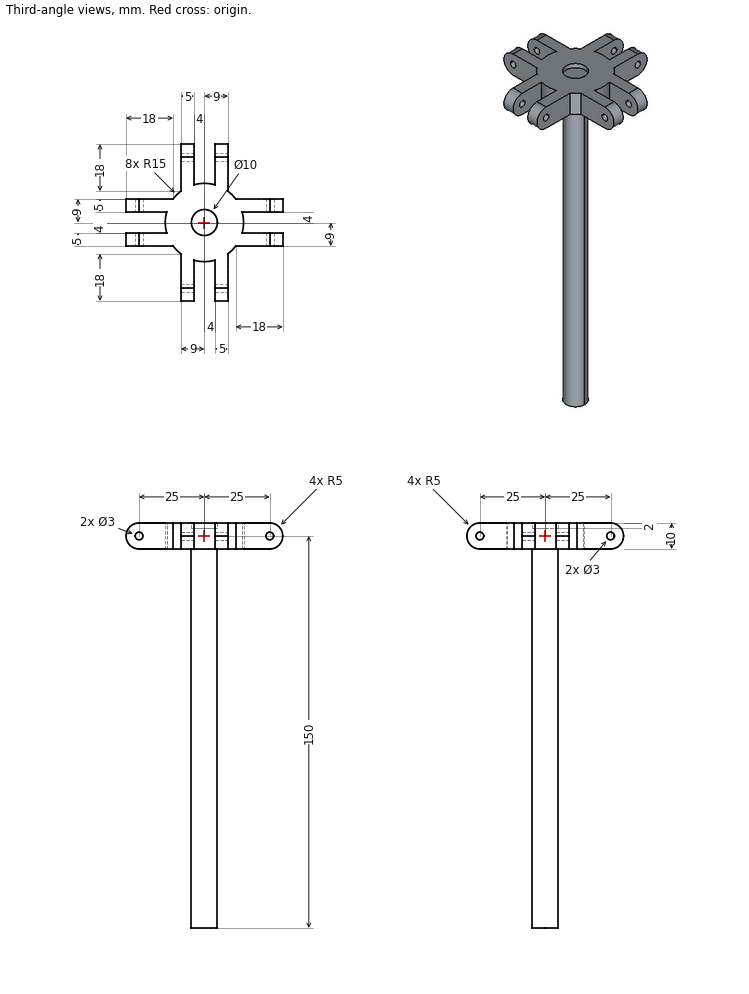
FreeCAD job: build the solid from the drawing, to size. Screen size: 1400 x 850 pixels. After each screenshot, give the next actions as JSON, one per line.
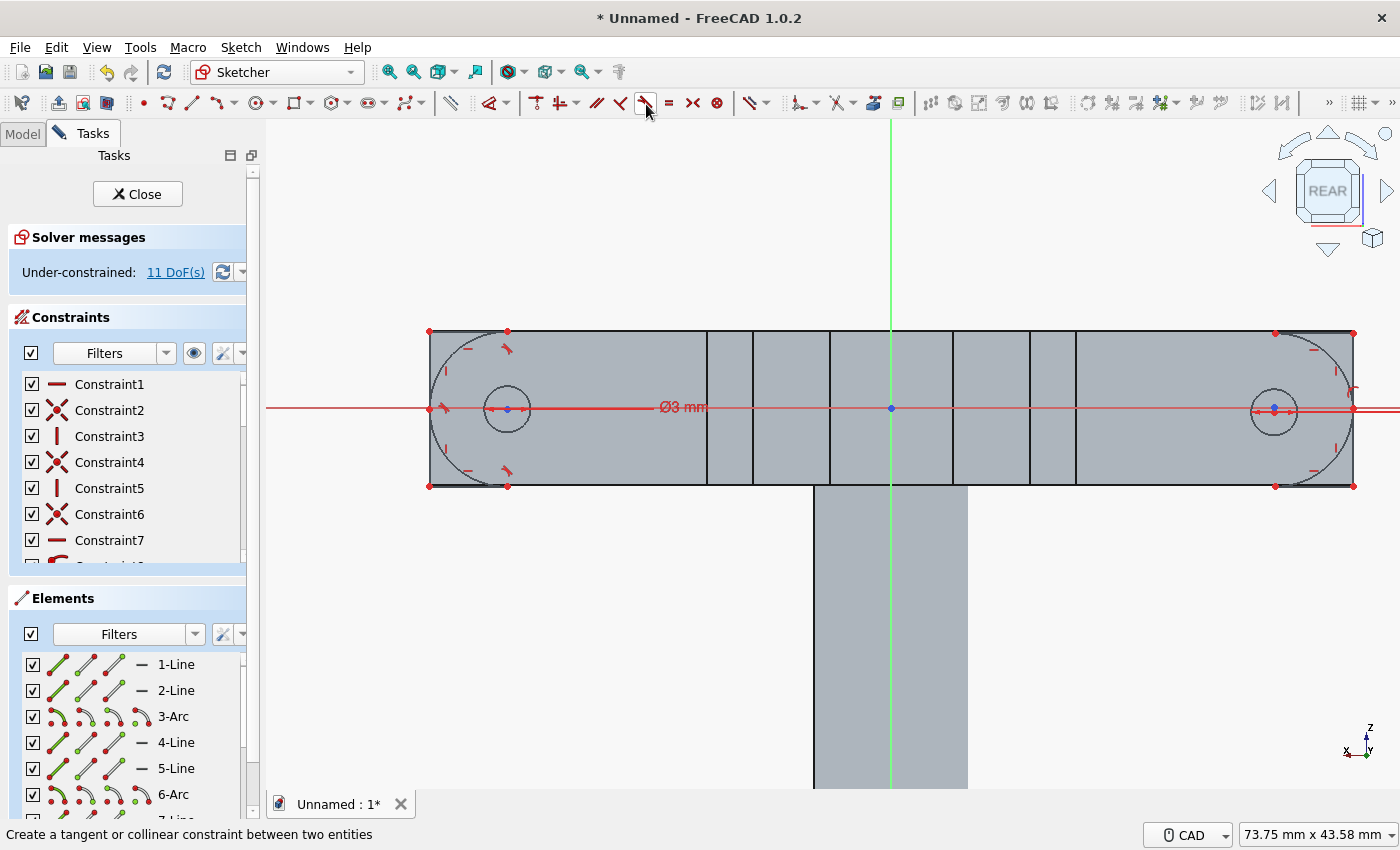
{"action": "scroll", "coordinate": [507, 547], "scroll_direction": "down", "scroll_amount": 2}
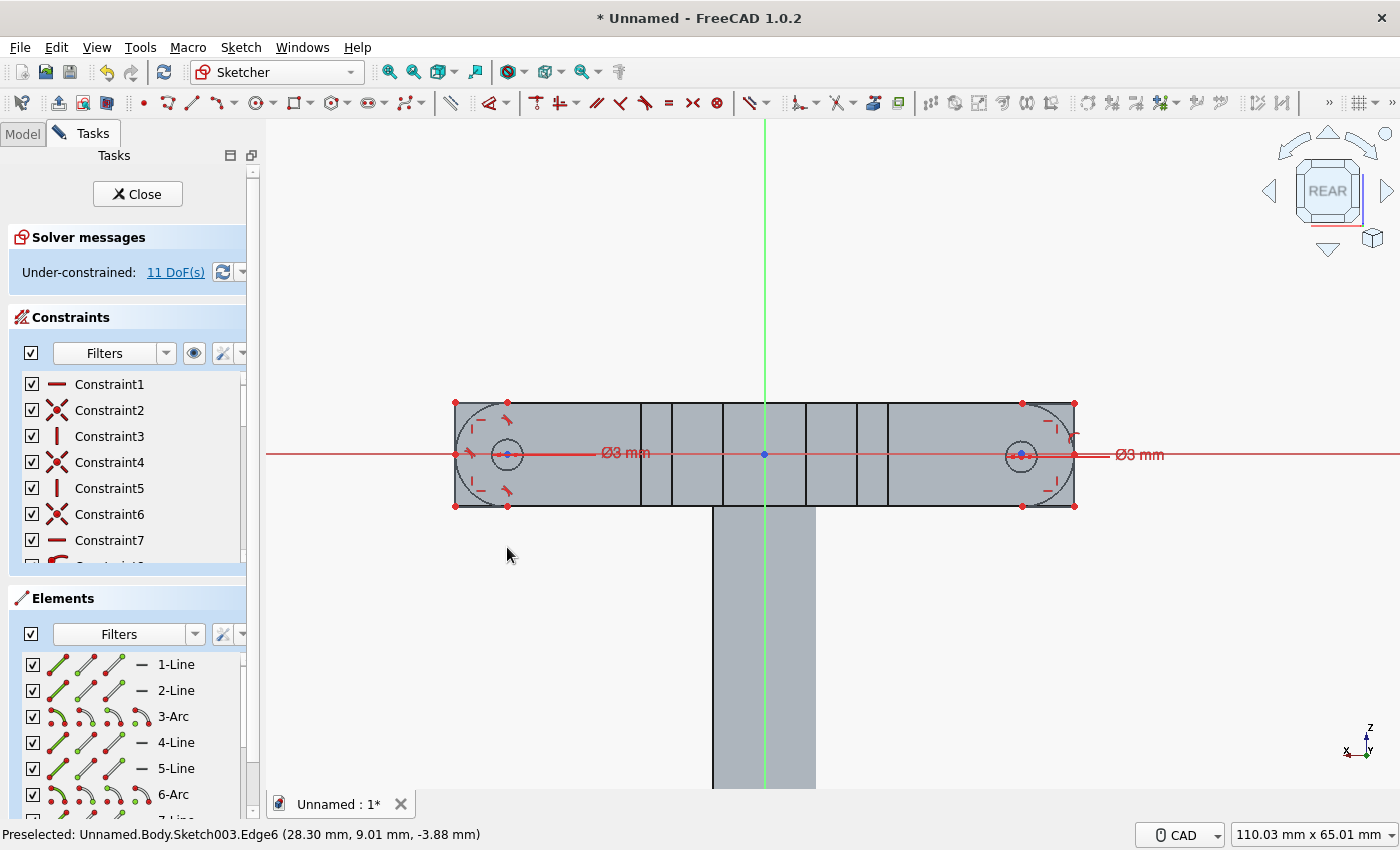
{"action": "left_click", "coordinate": [1074, 419]}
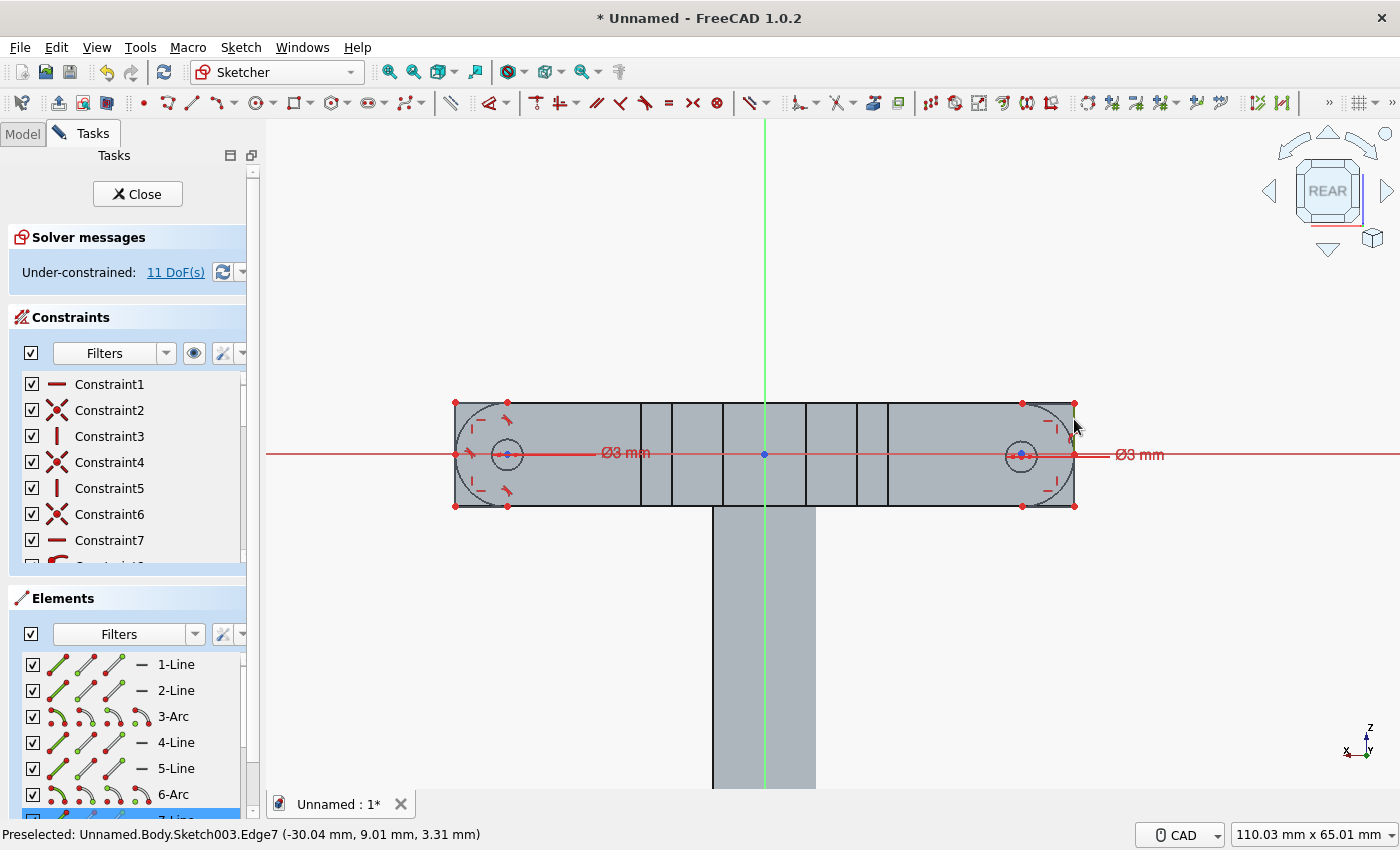
{"action": "left_click", "coordinate": [1058, 419]}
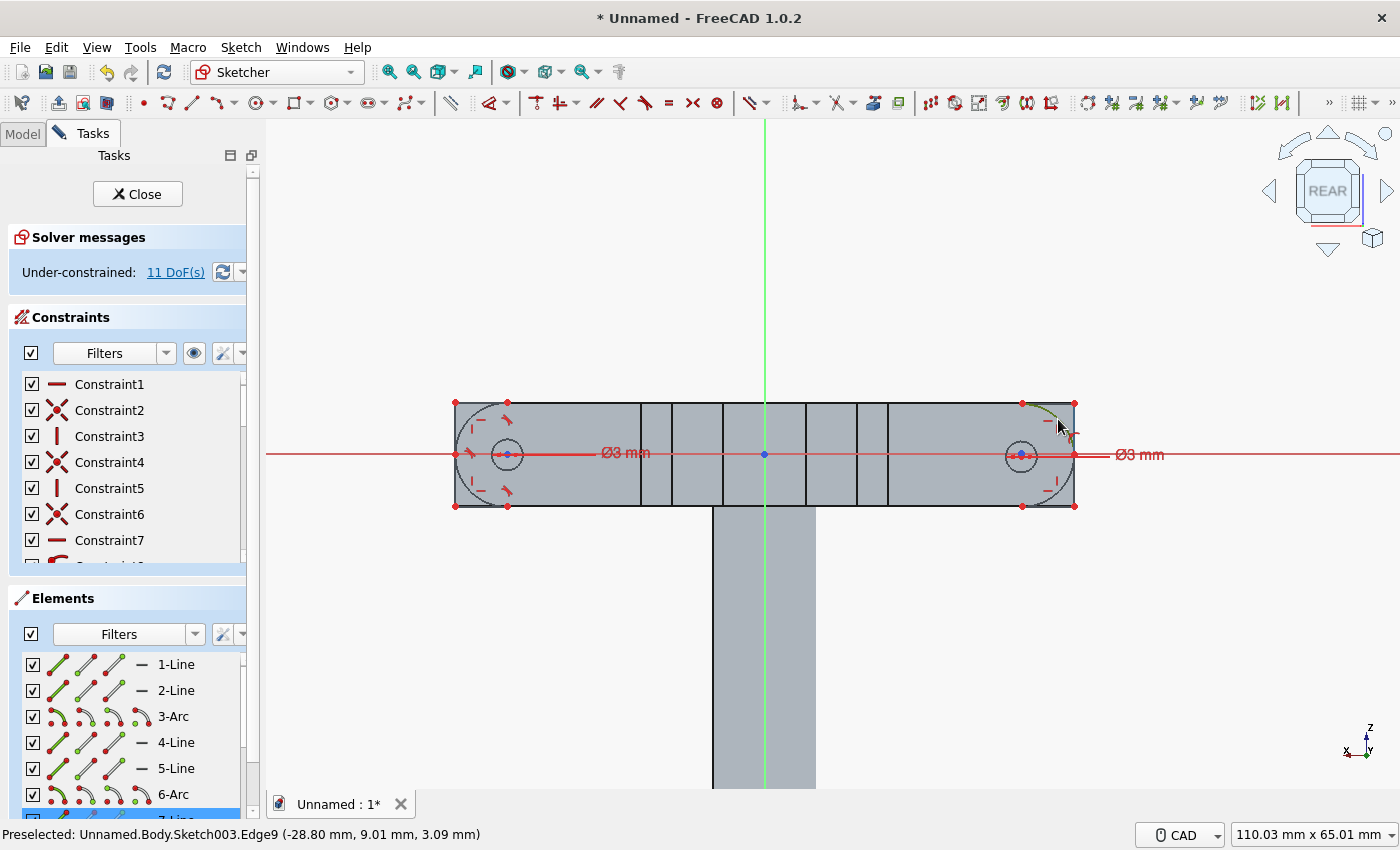
{"action": "key", "text": "t"}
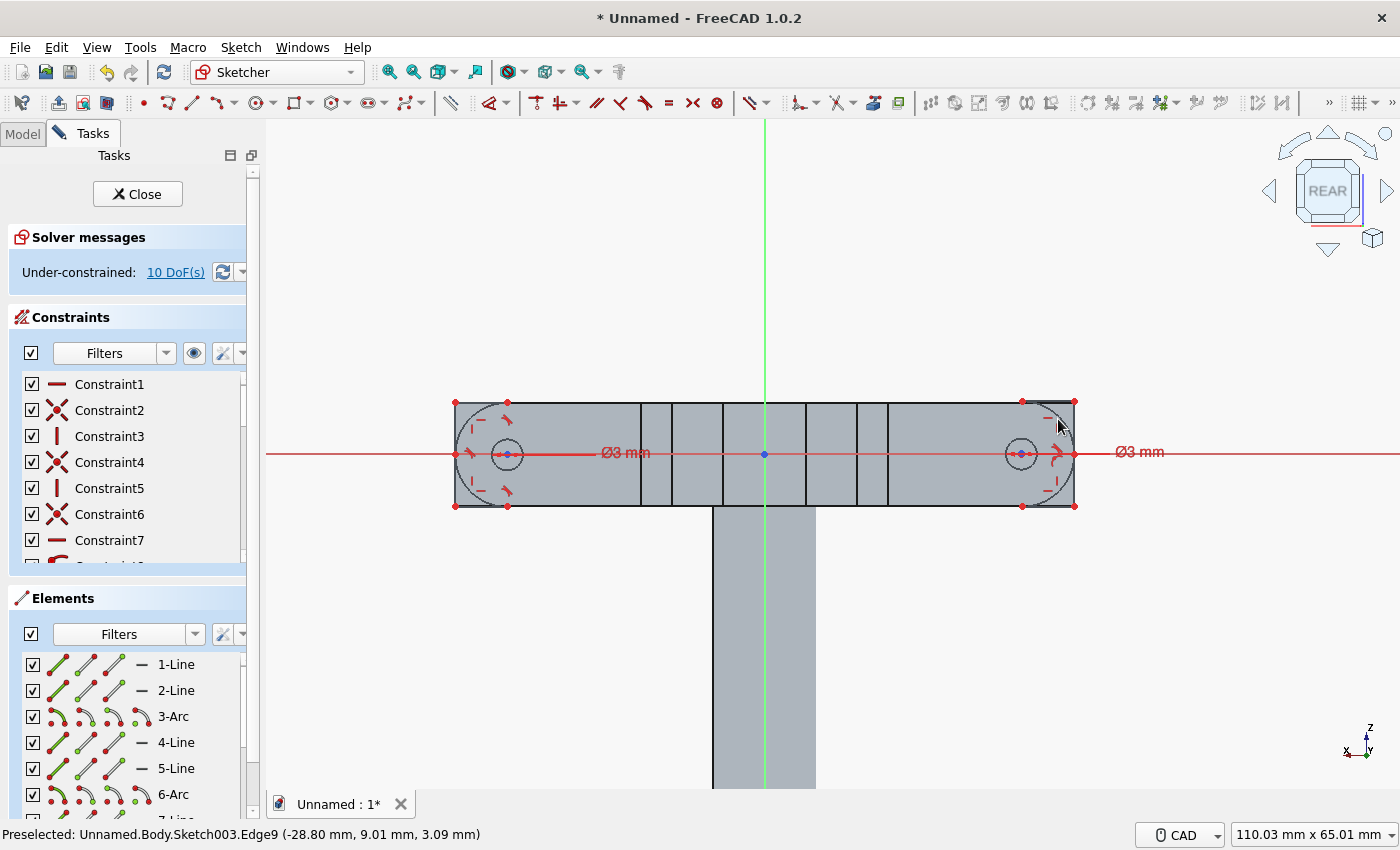
{"action": "left_click", "coordinate": [1074, 417]}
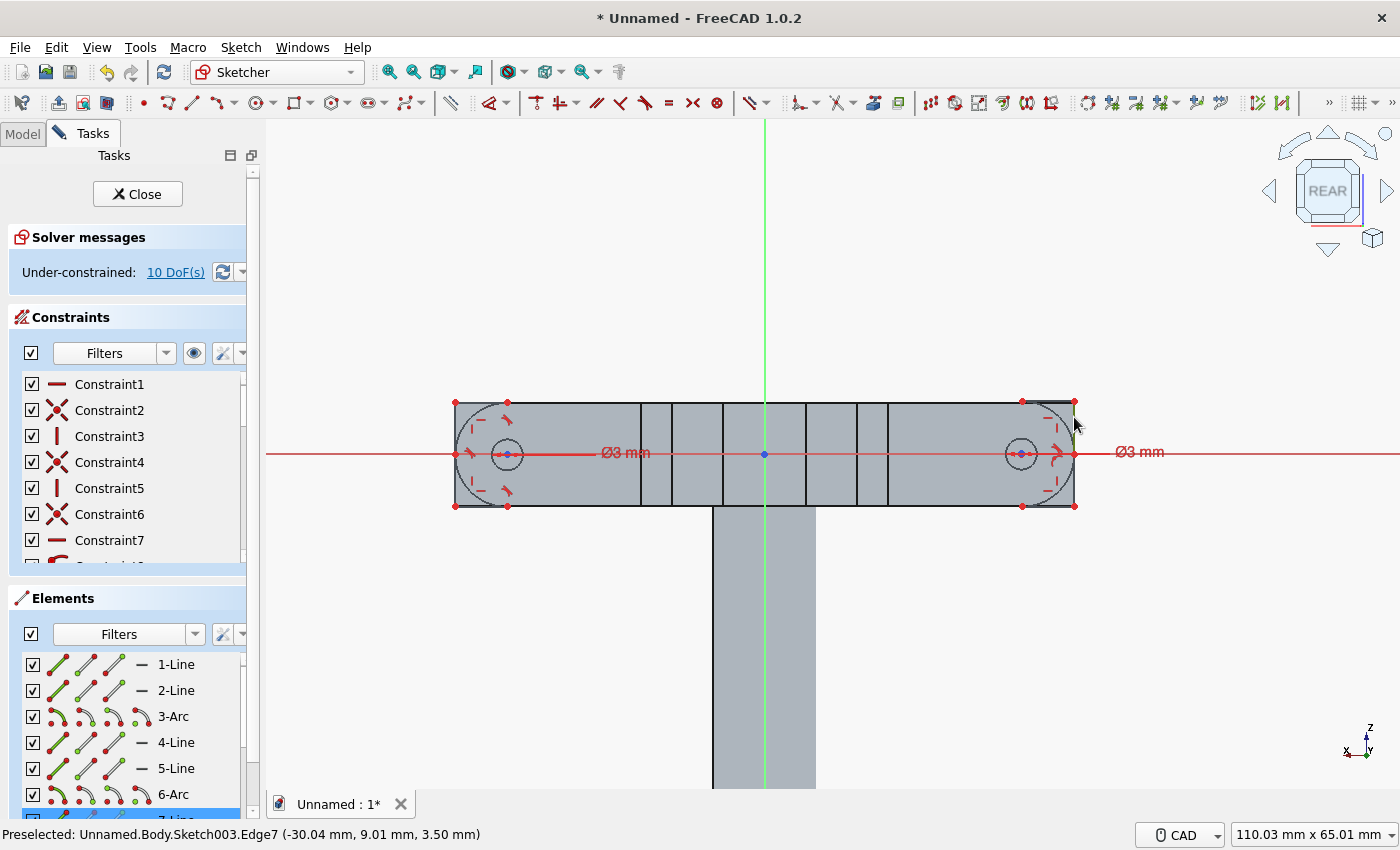
{"action": "left_click", "coordinate": [1059, 491]}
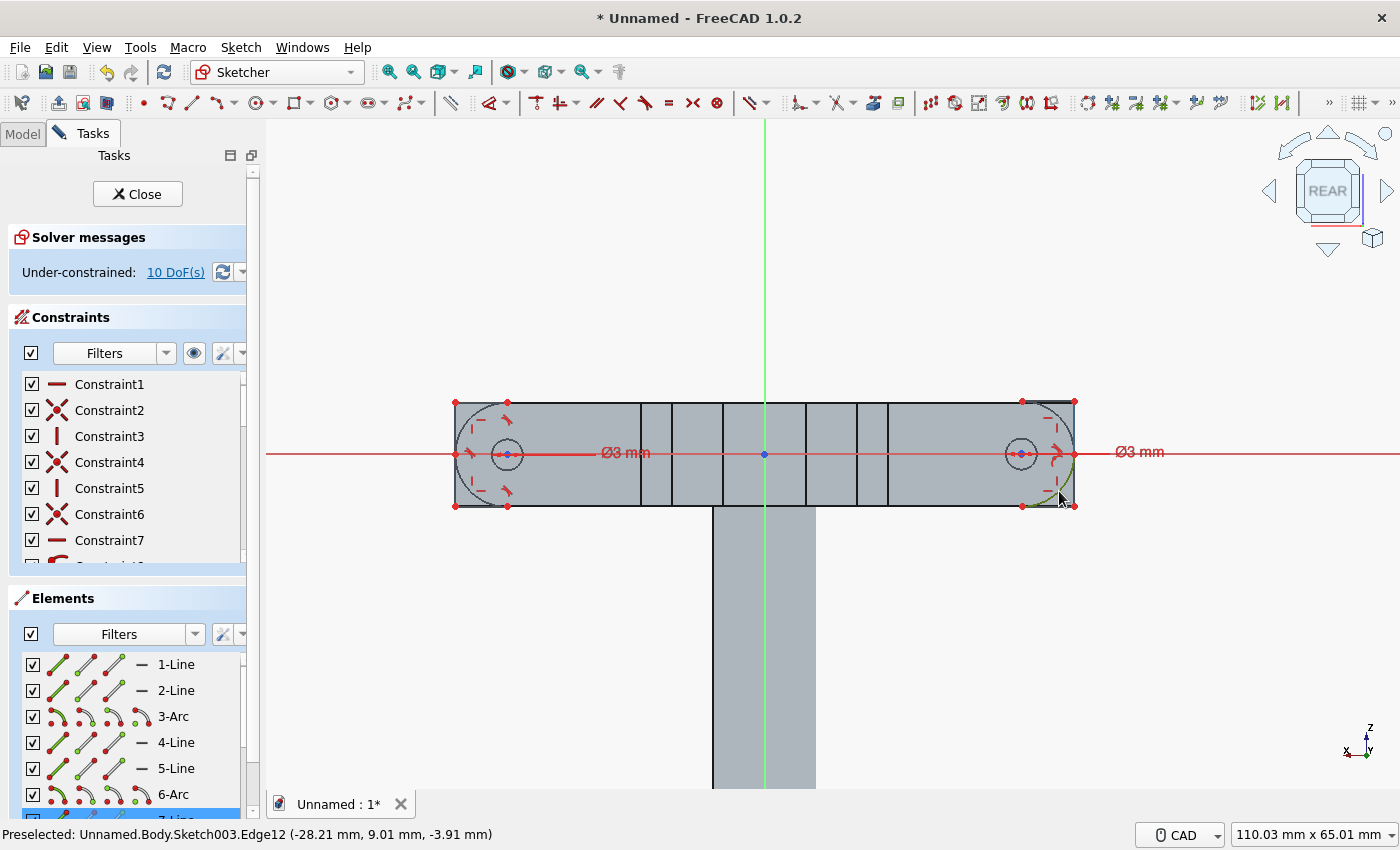
{"action": "key", "text": "t"}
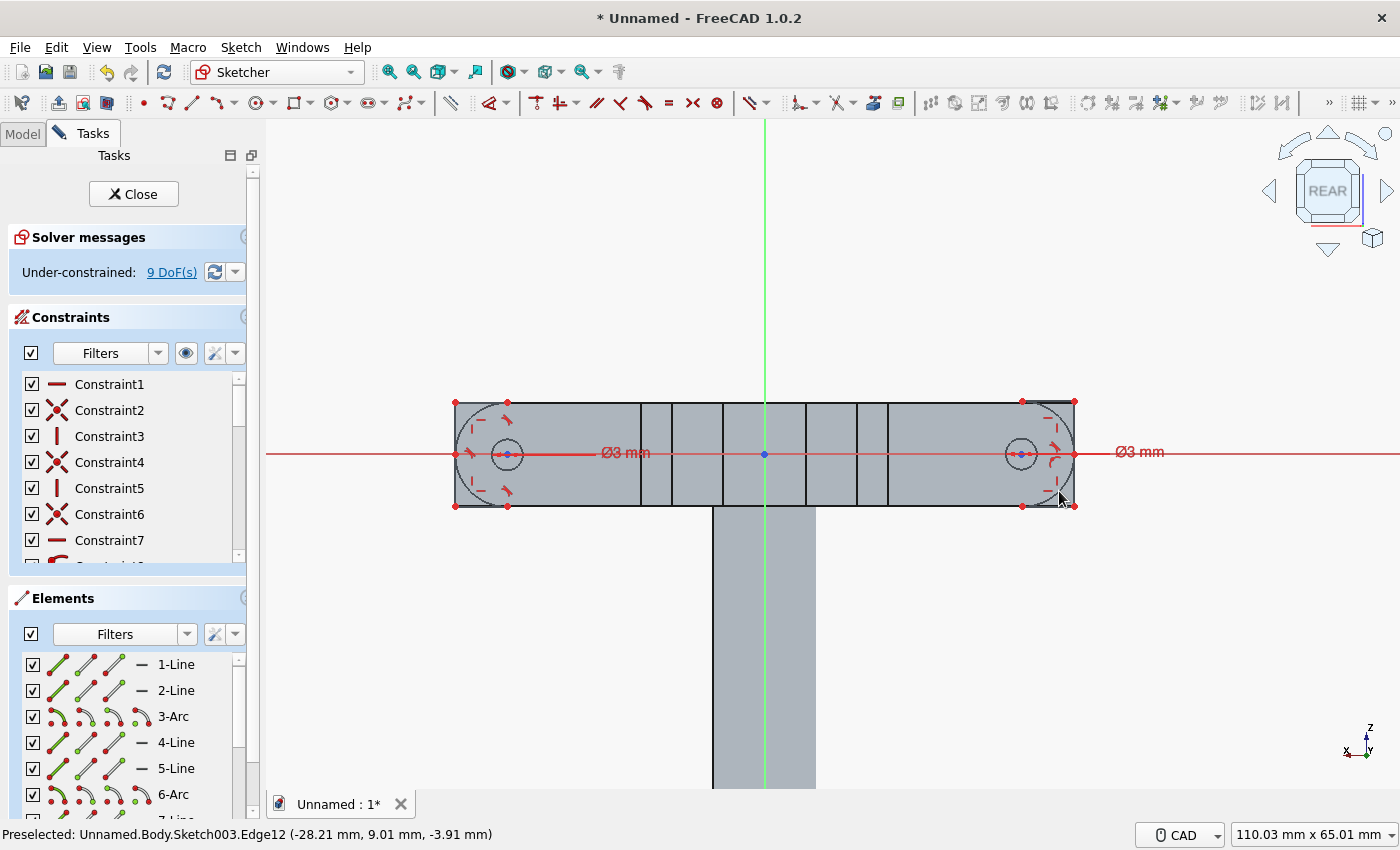
{"action": "left_click", "coordinate": [1059, 401]}